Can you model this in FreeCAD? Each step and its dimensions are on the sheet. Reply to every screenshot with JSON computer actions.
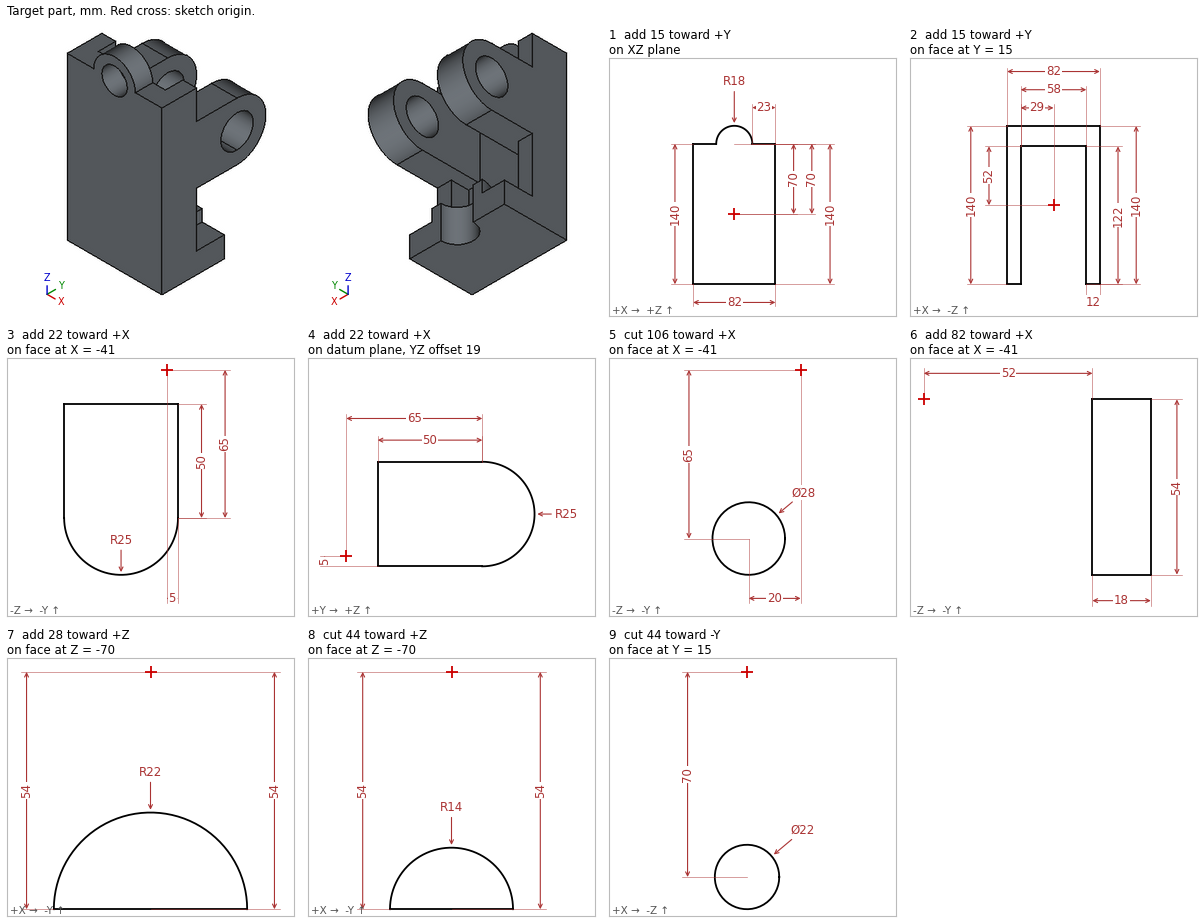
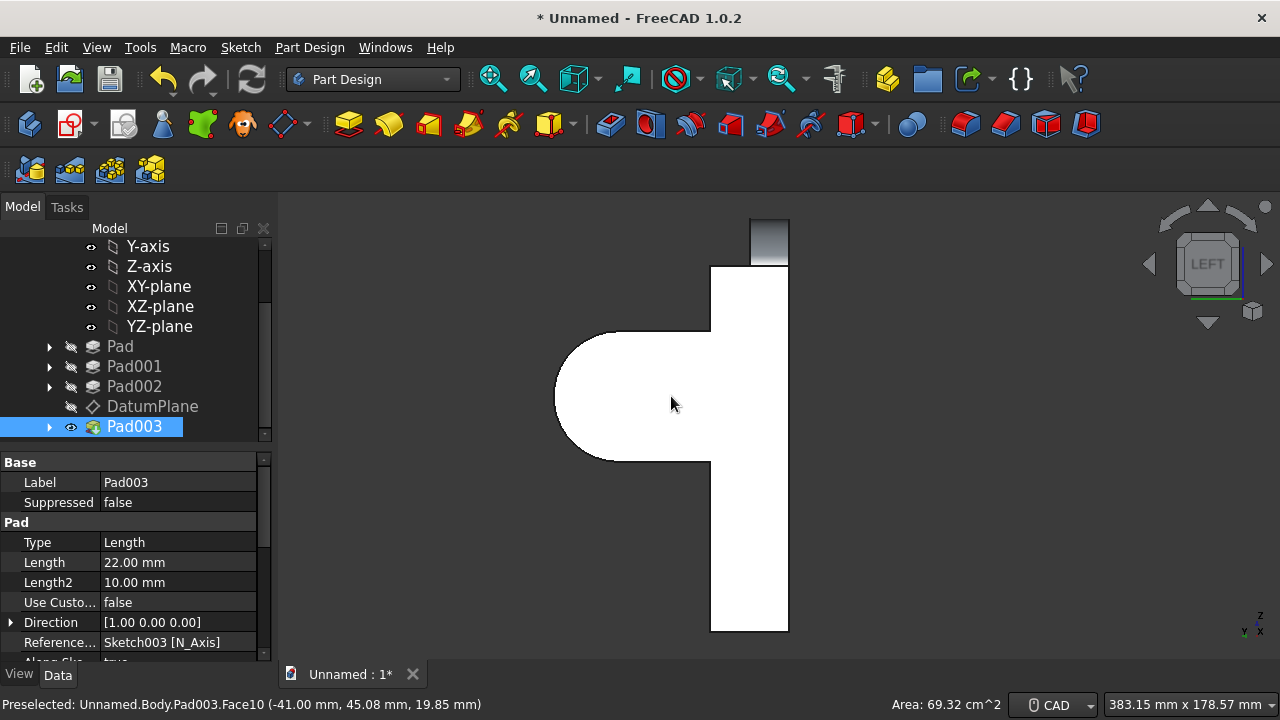
{"action": "left_click", "coordinate": [70, 124]}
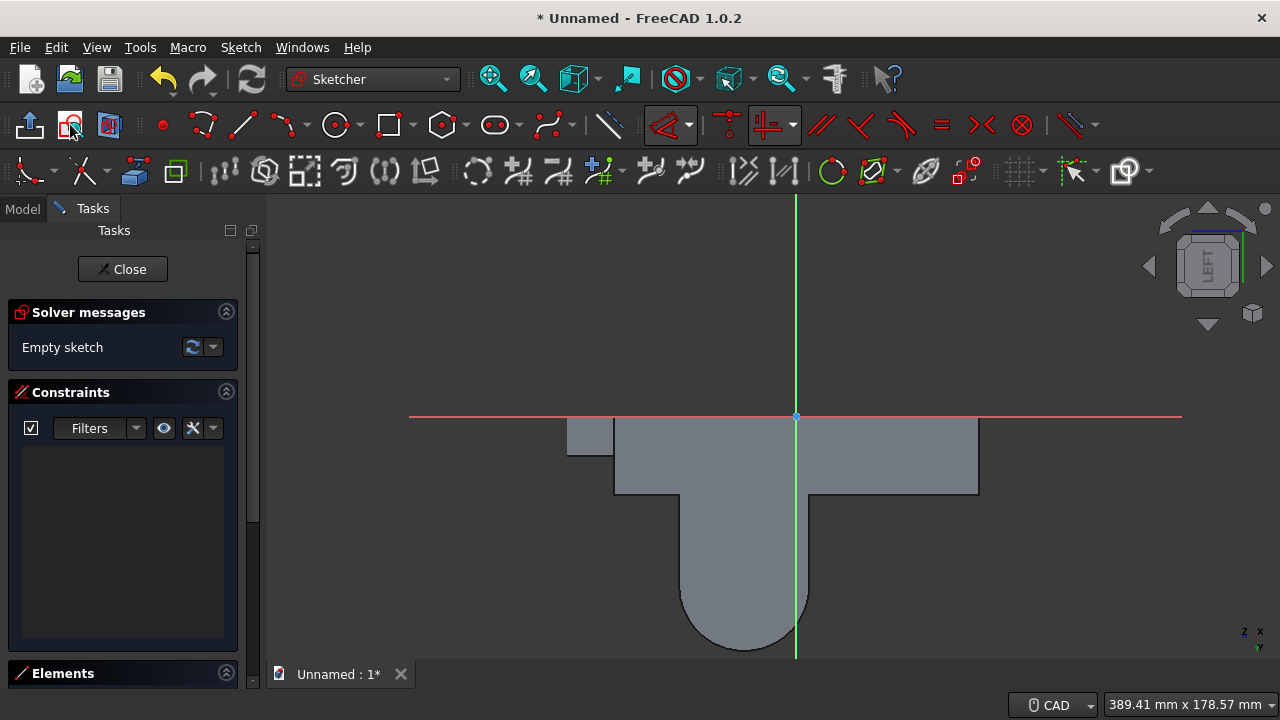
{"action": "scroll", "coordinate": [757, 631], "scroll_direction": "up", "scroll_amount": 7}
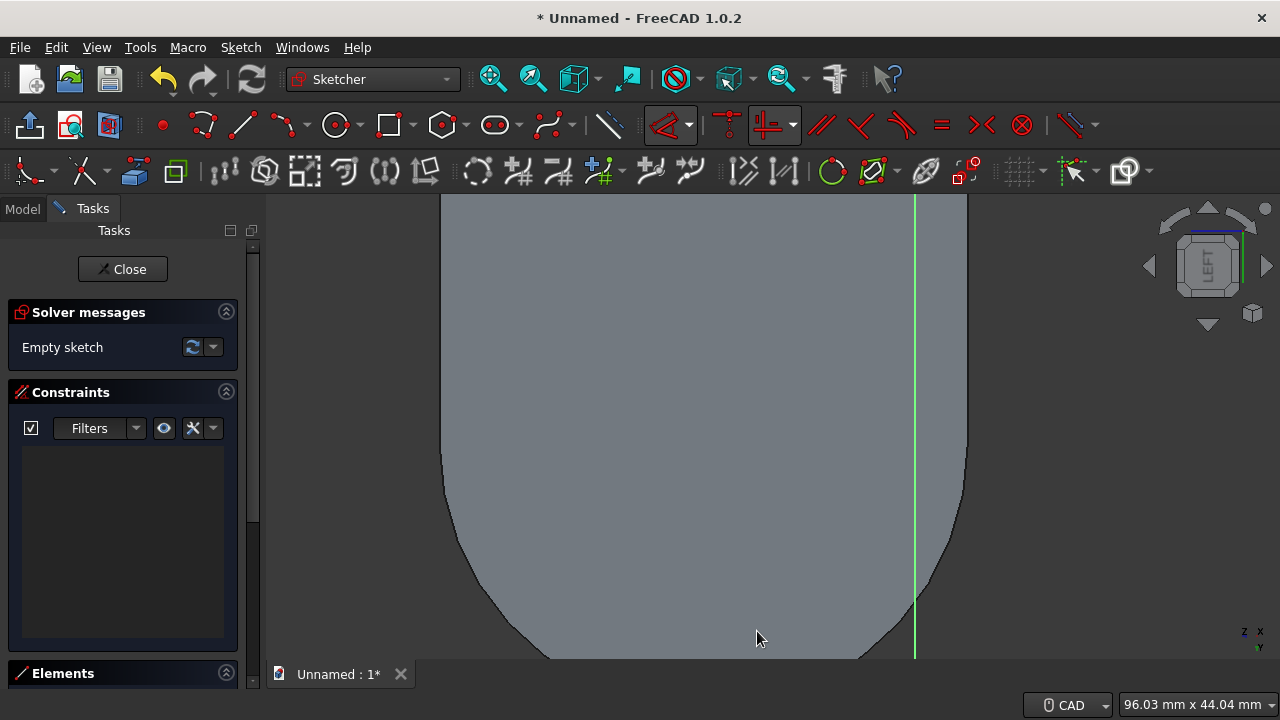
{"action": "key", "text": "g c"}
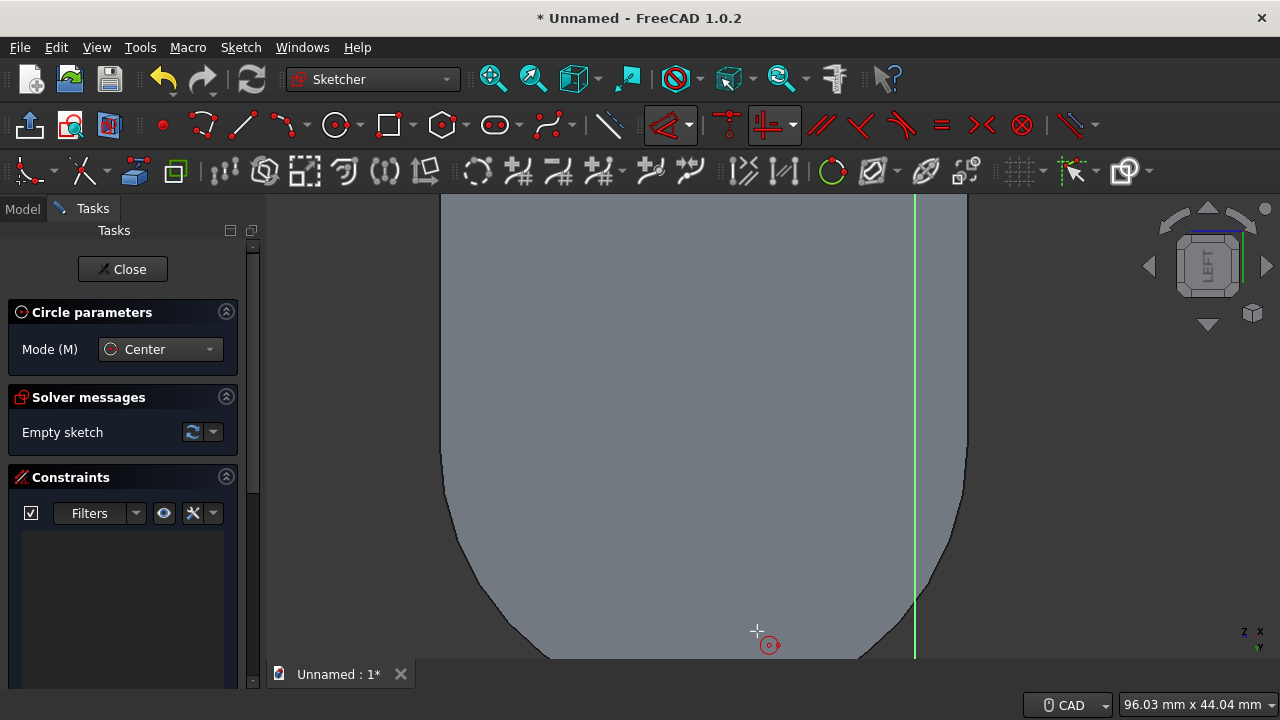
{"action": "left_click", "coordinate": [704, 445]}
{"action": "mouse_move", "coordinate": [808, 341]}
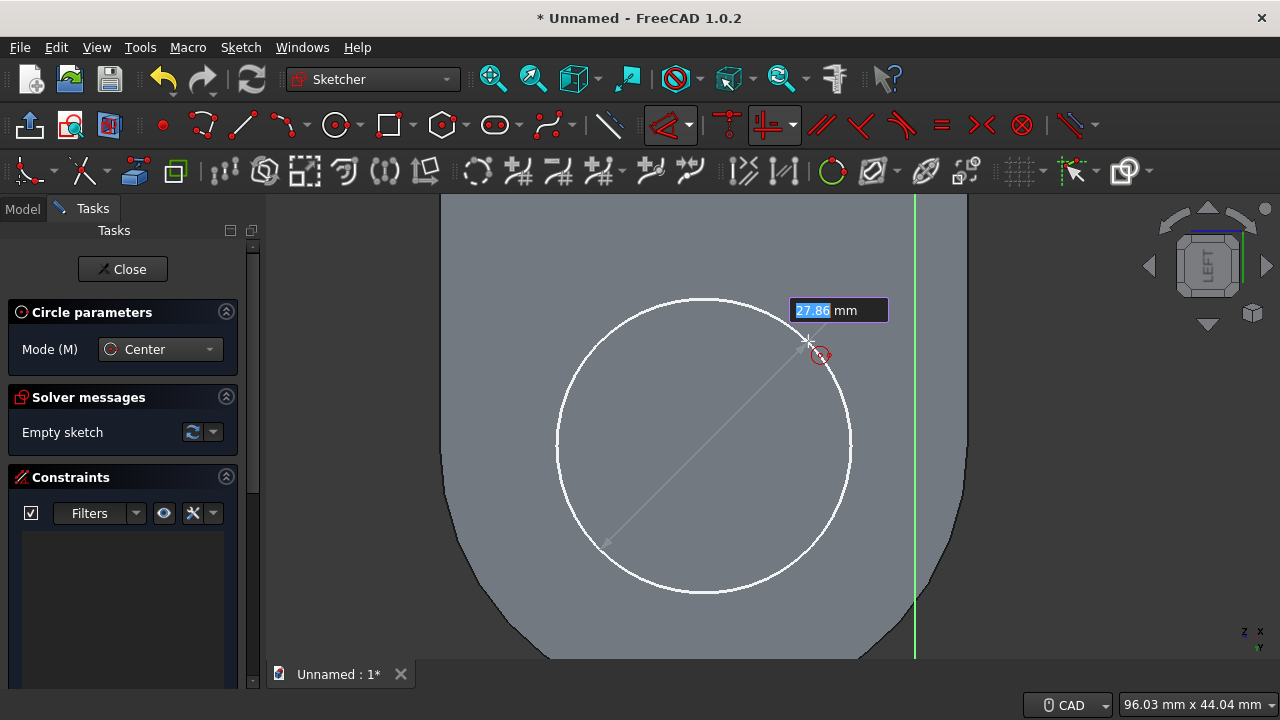
{"action": "type", "text": "28"}
{"action": "key", "text": "Return"}
{"action": "key", "text": "Escape"}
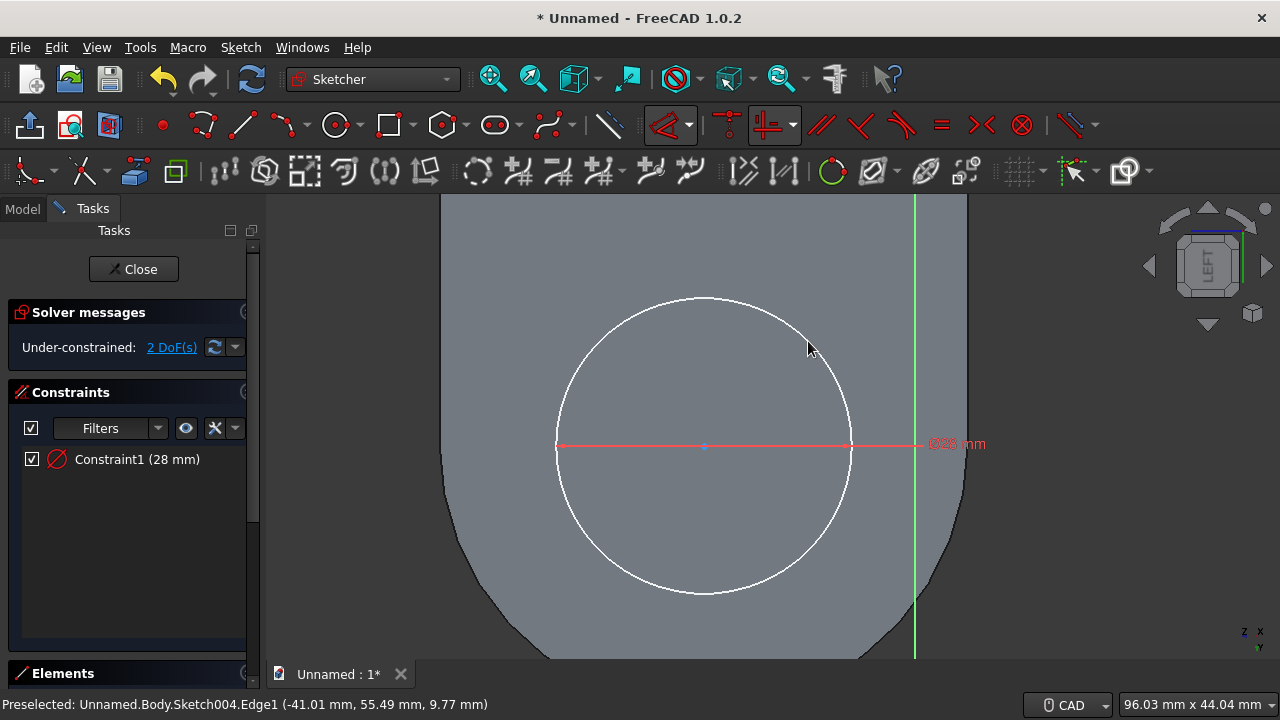
{"action": "left_click", "coordinate": [704, 446]}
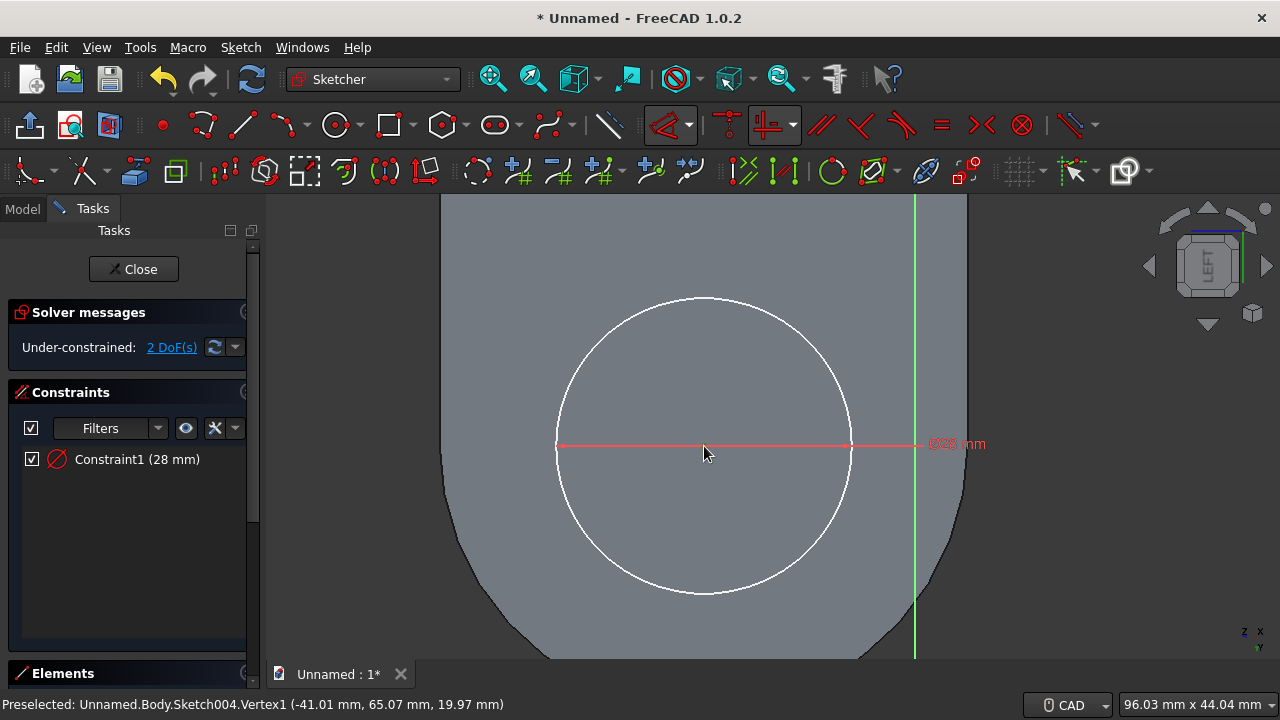
{"action": "key", "text": "l"}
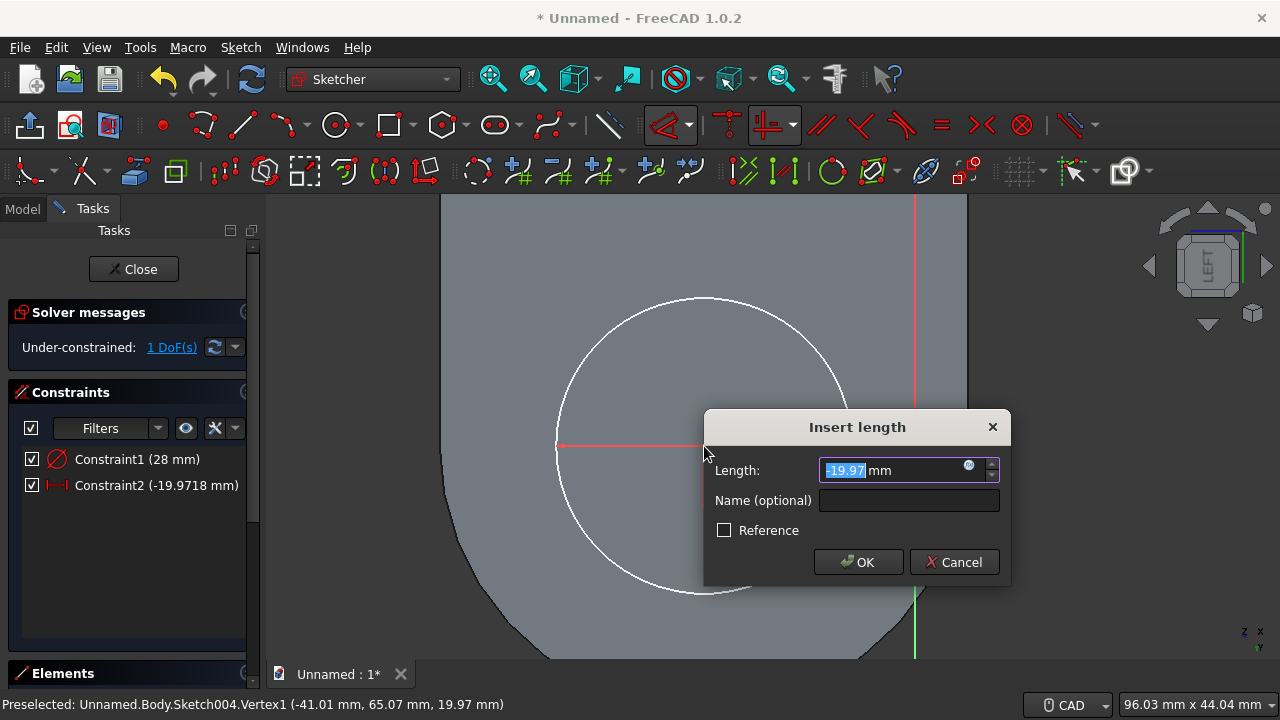
{"action": "type", "text": "-20"}
{"action": "key", "text": "Return"}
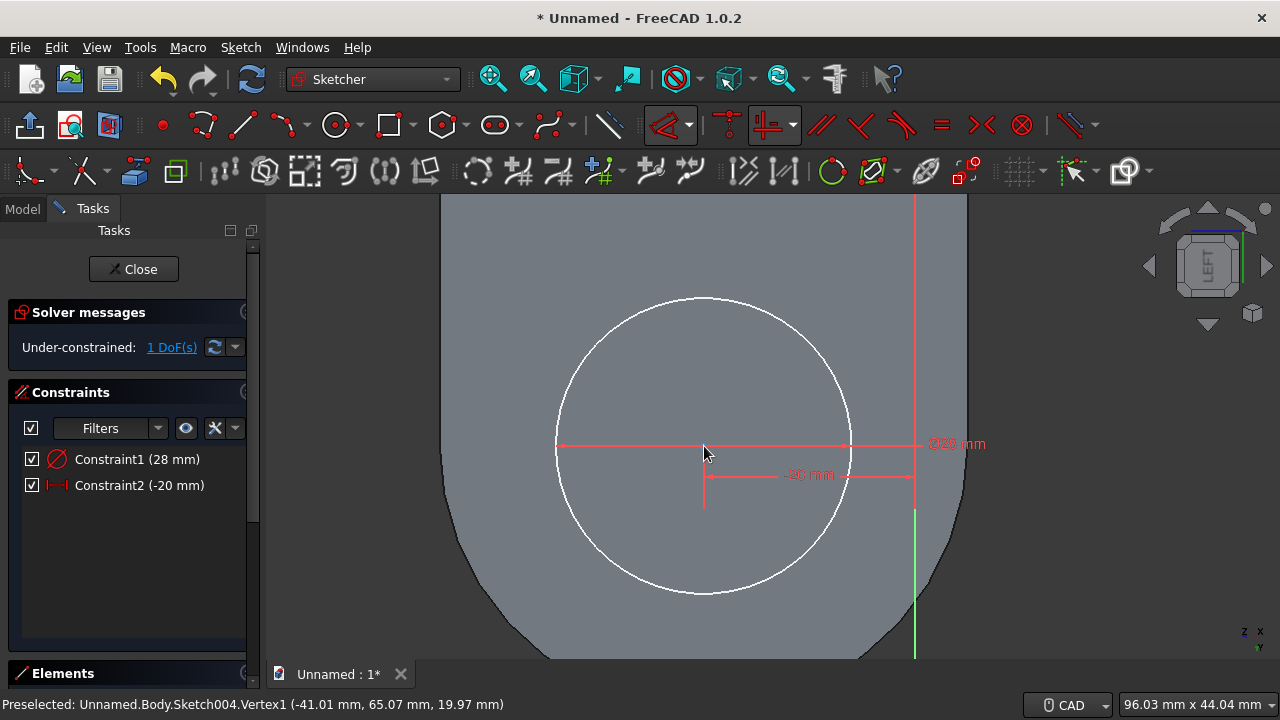
{"action": "left_click", "coordinate": [704, 446]}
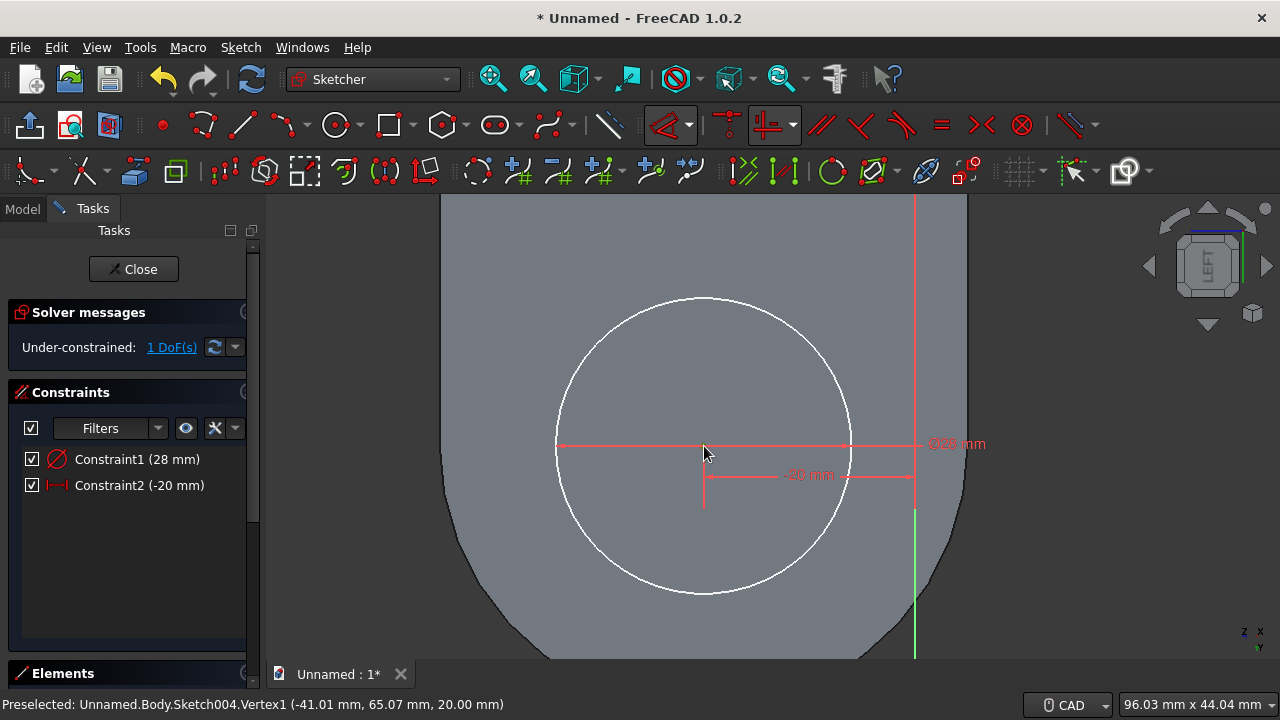
{"action": "key", "text": "i"}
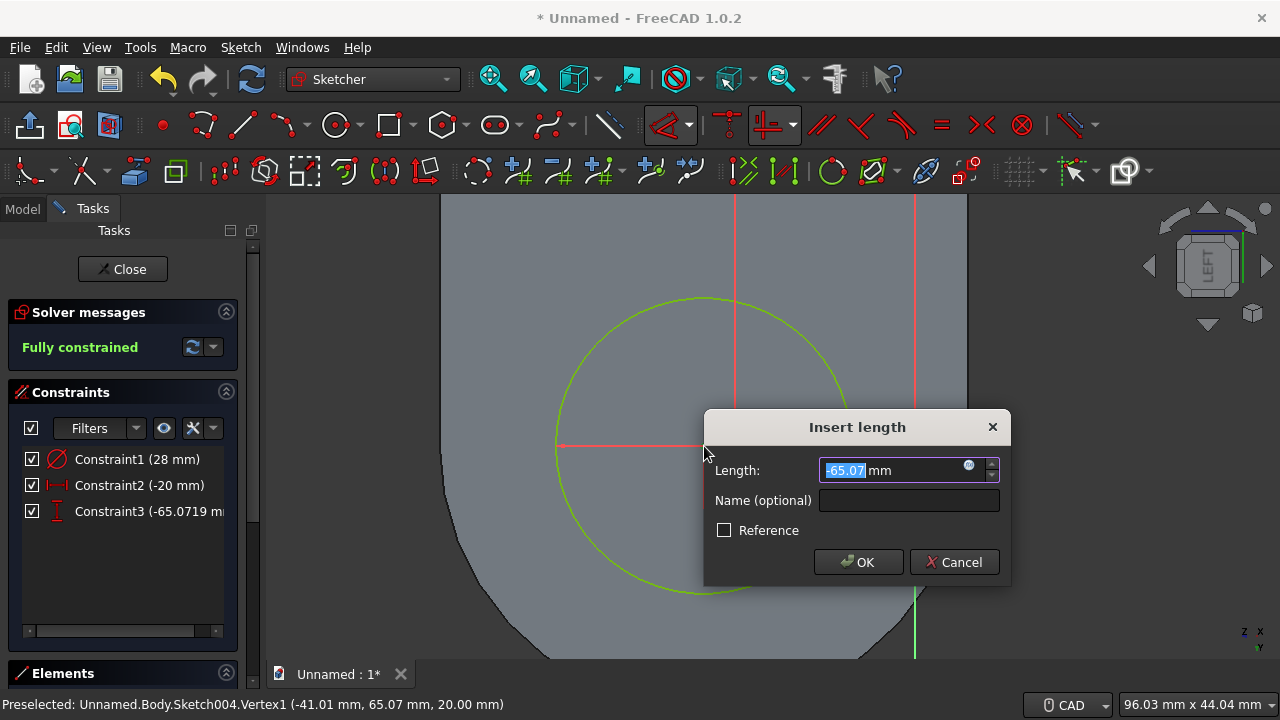
{"action": "type", "text": "-65"}
{"action": "key", "text": "Return"}